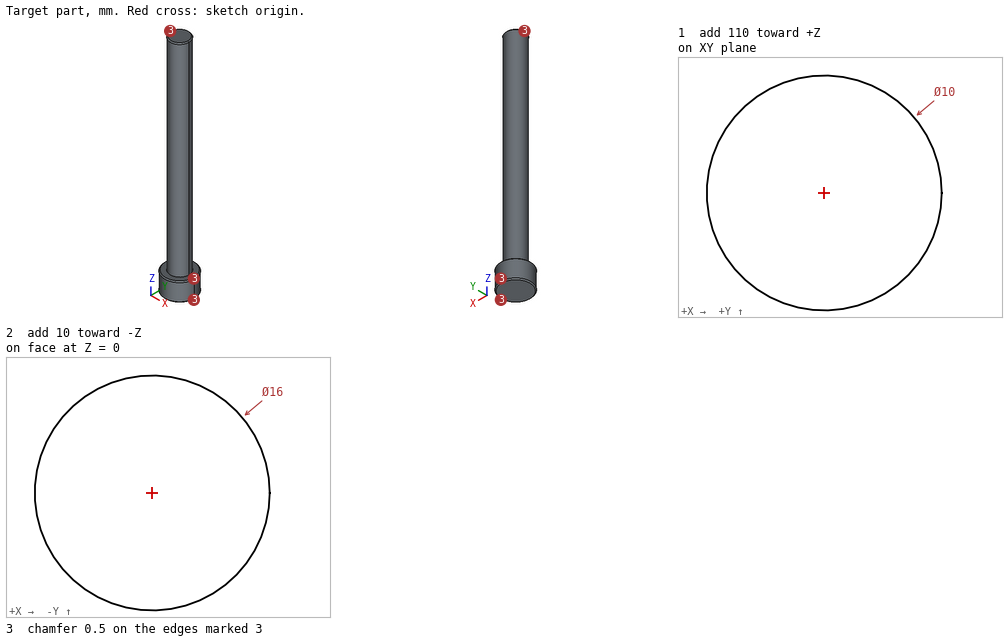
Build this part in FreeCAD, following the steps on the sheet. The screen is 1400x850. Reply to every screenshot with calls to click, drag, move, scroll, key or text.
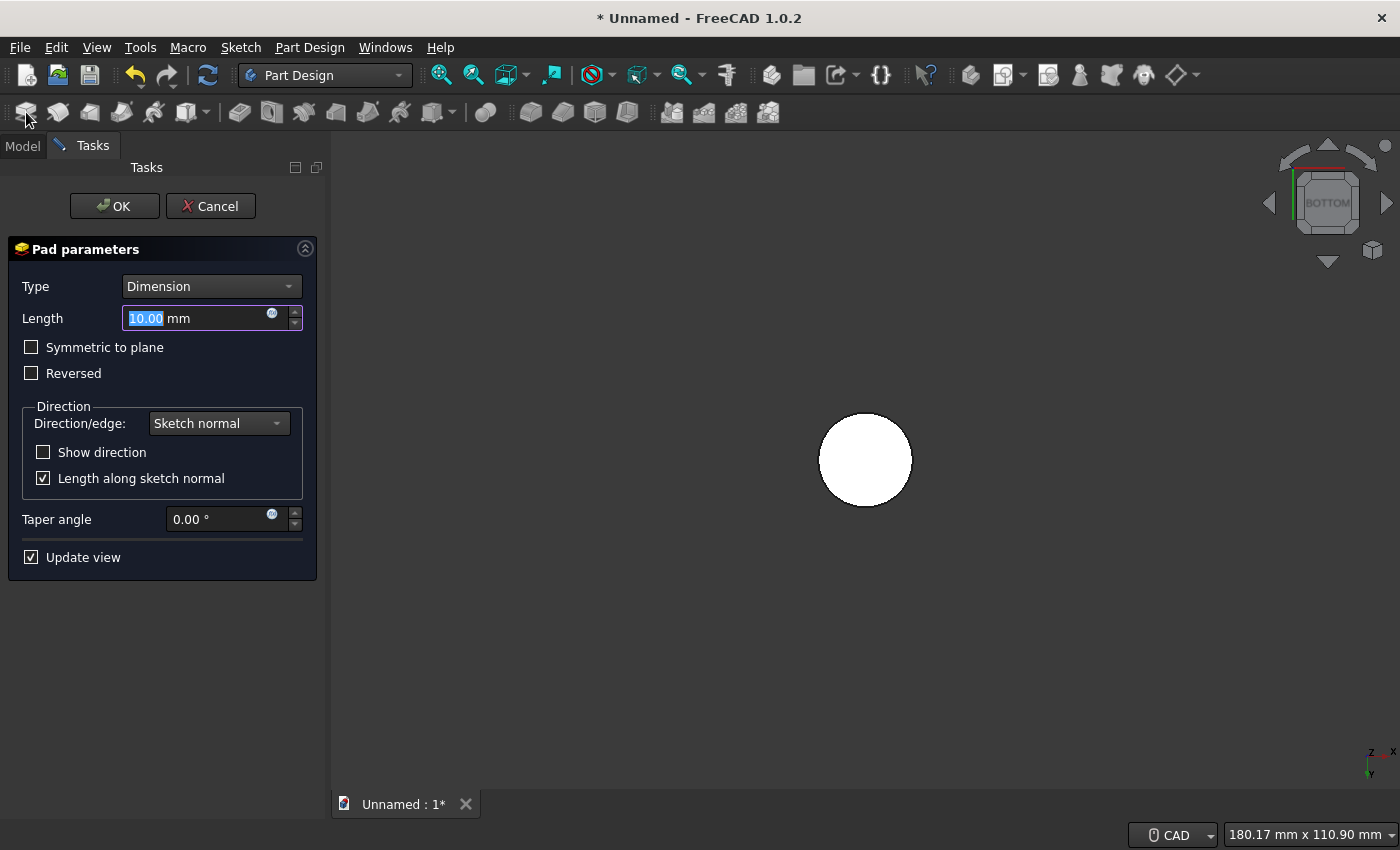
text(10)
key(Tab)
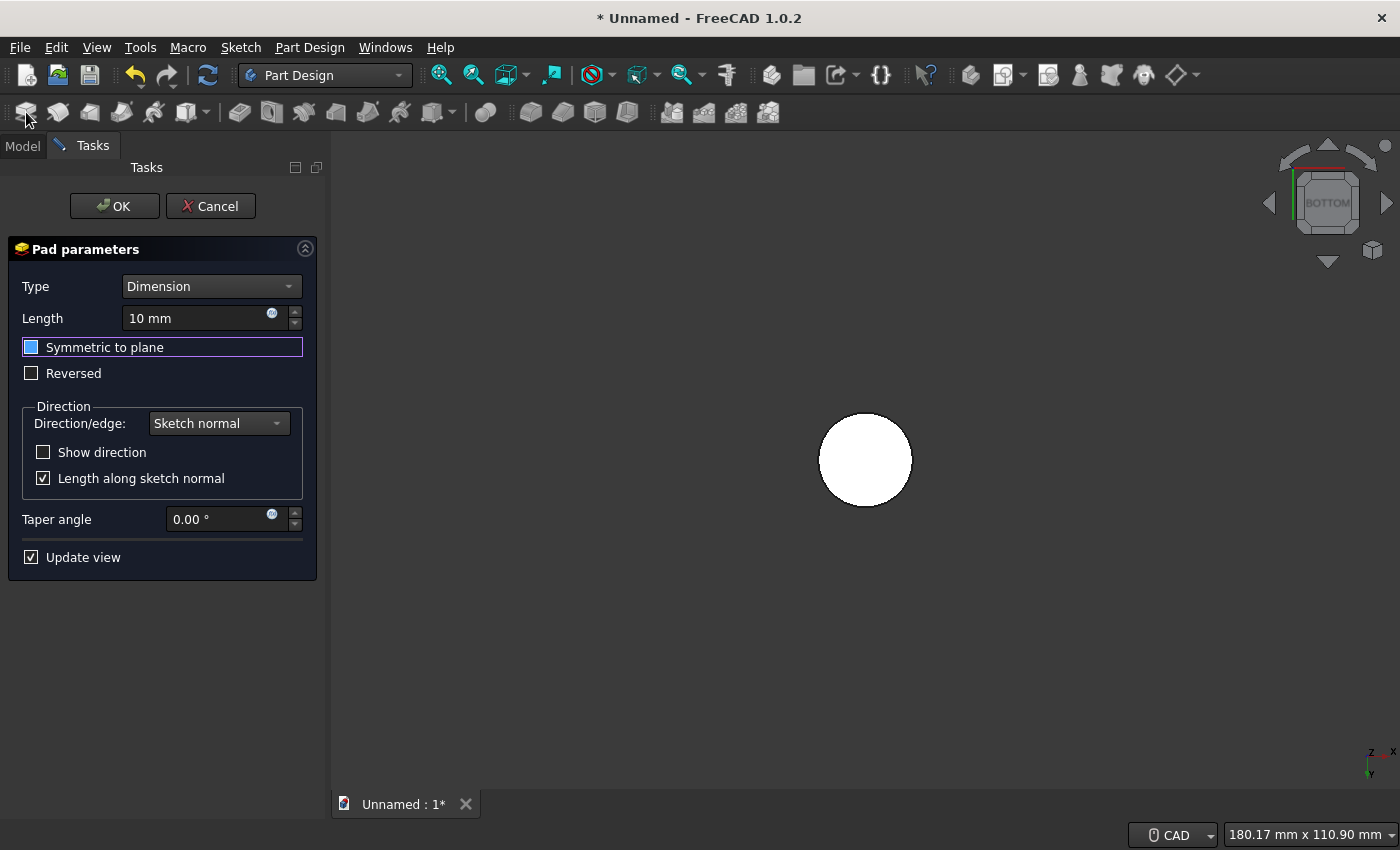
click(115, 206)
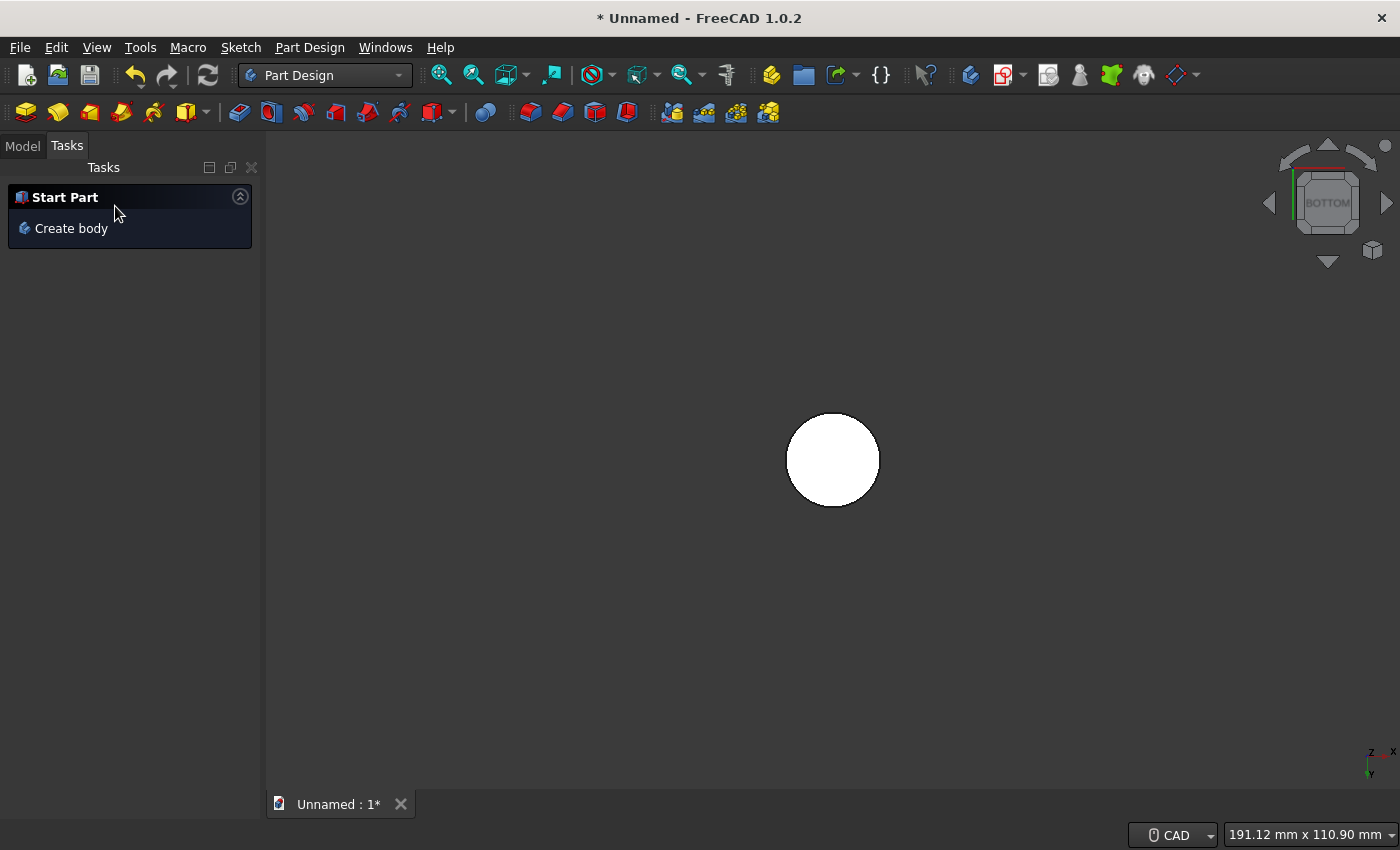
click(442, 76)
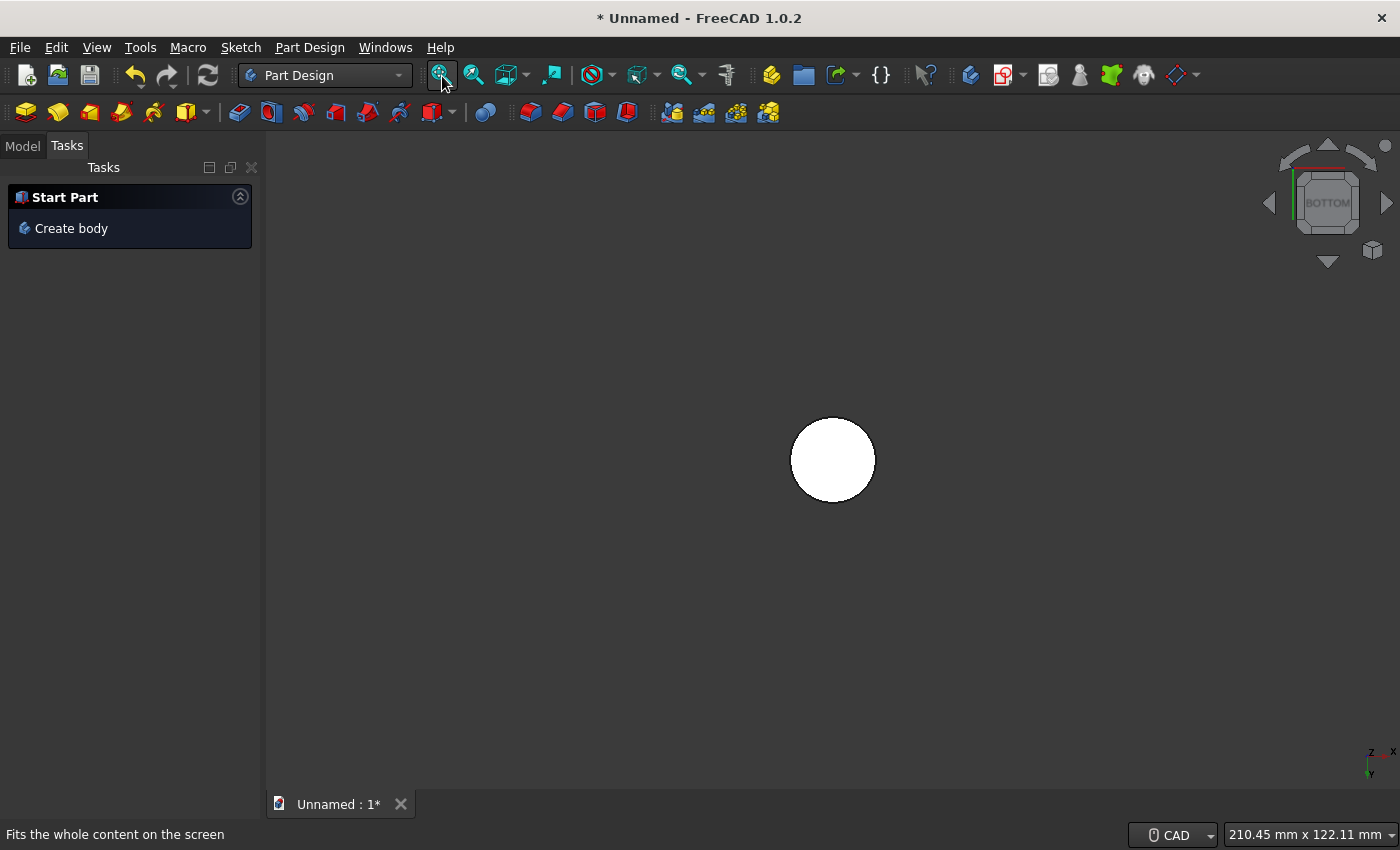
click(790, 459)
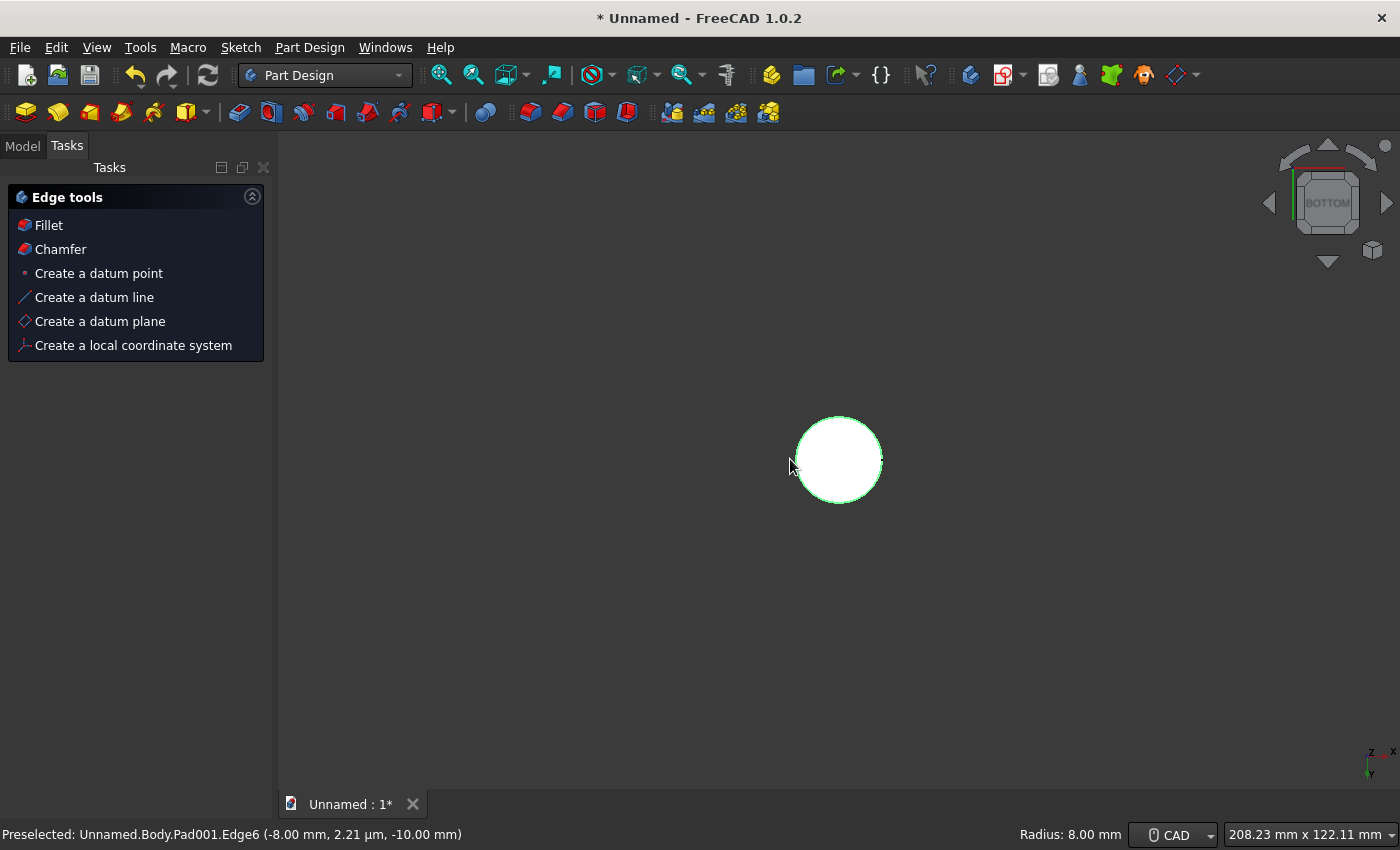
key(0)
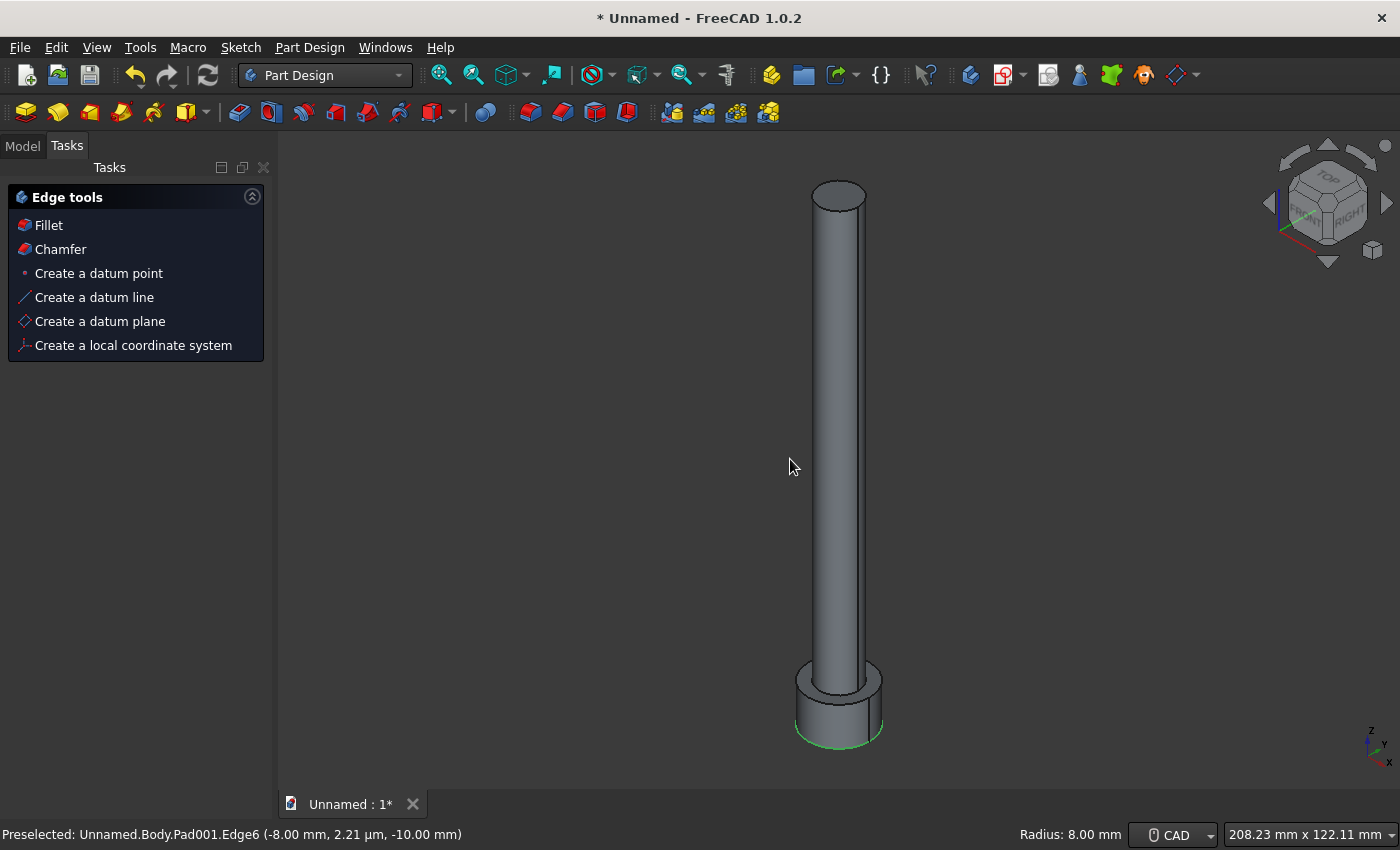
click(812, 193, ctrl)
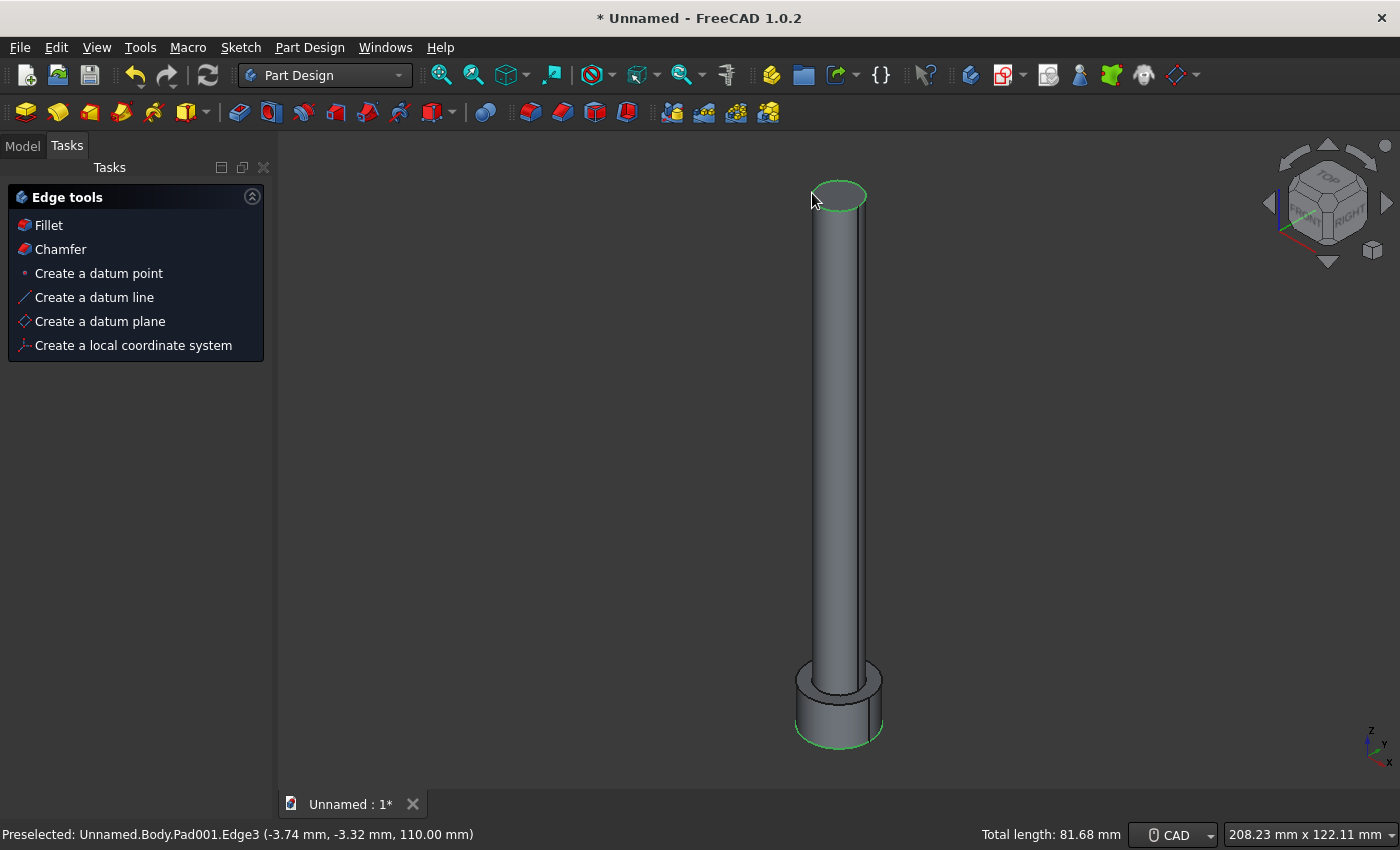
click(796, 675, ctrl)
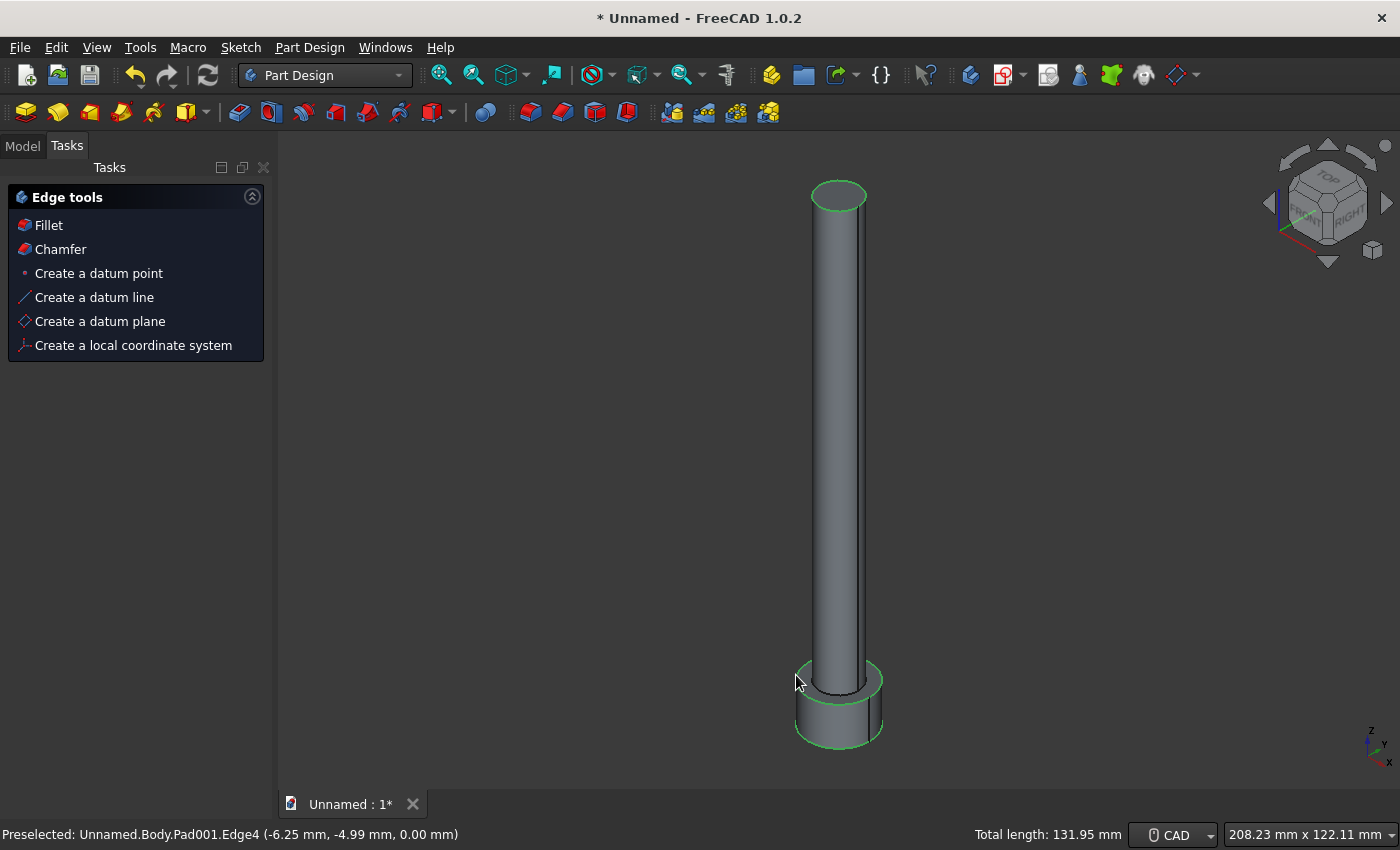
click(564, 112)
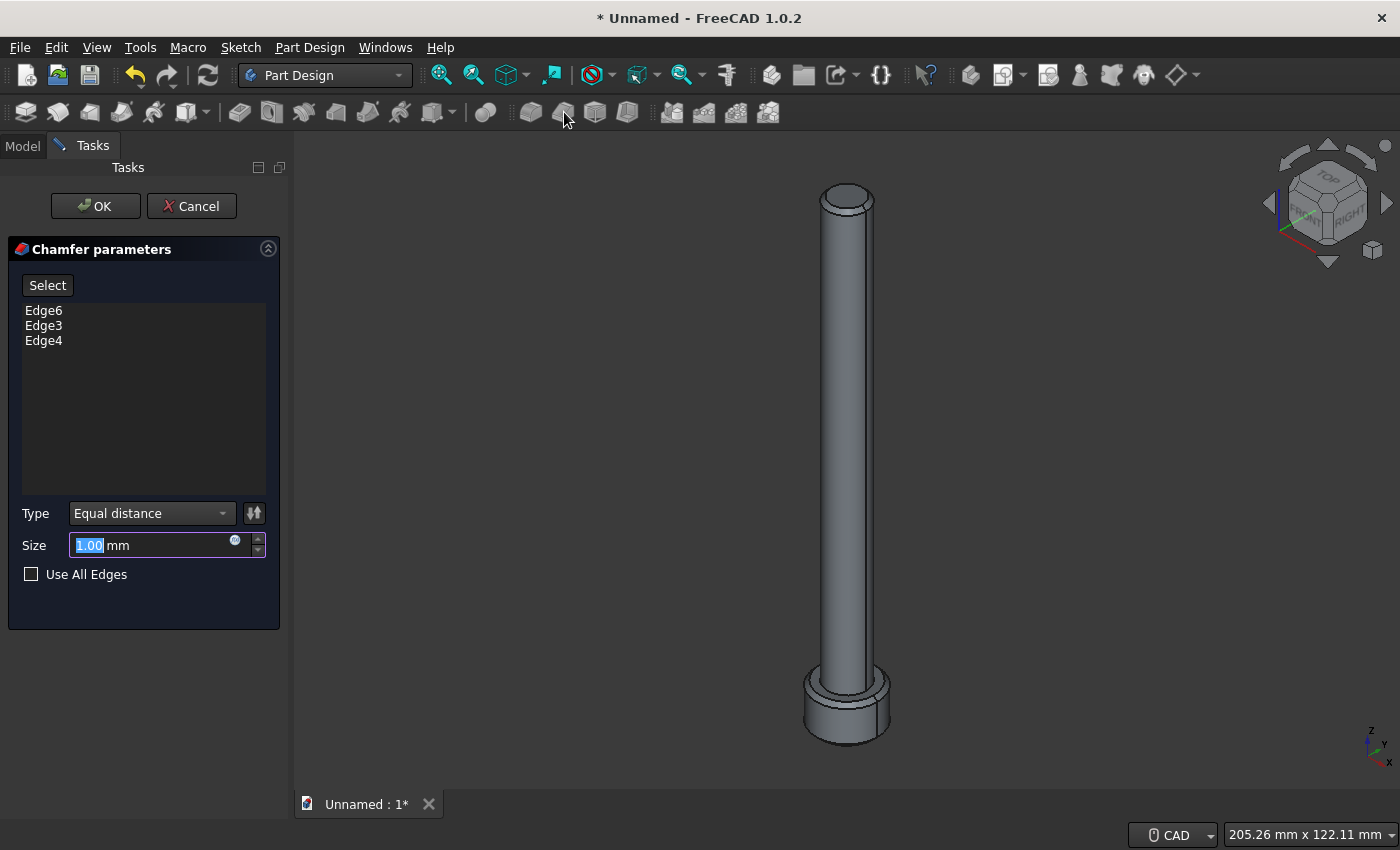
text(0.5)
key(Tab)